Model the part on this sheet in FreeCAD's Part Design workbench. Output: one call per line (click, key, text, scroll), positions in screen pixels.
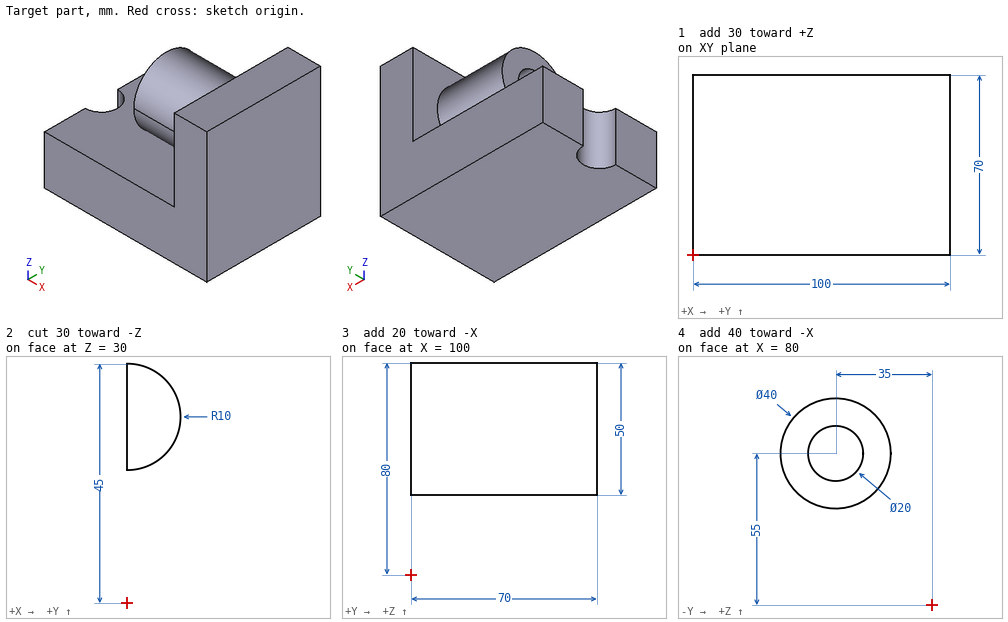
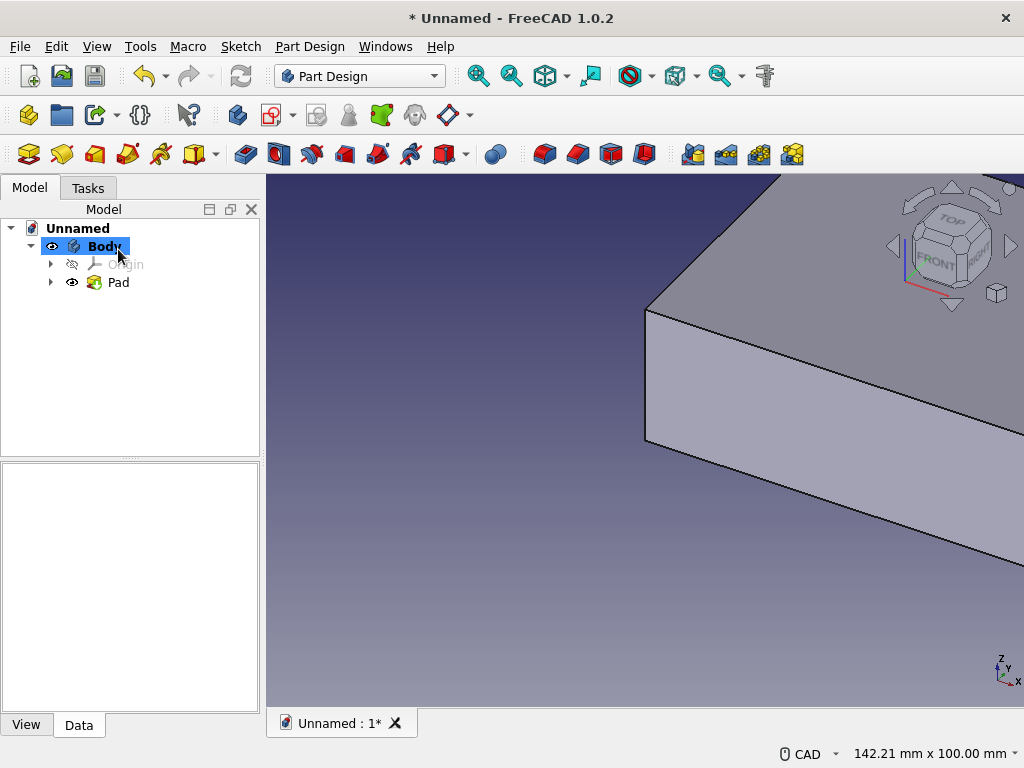
click(479, 76)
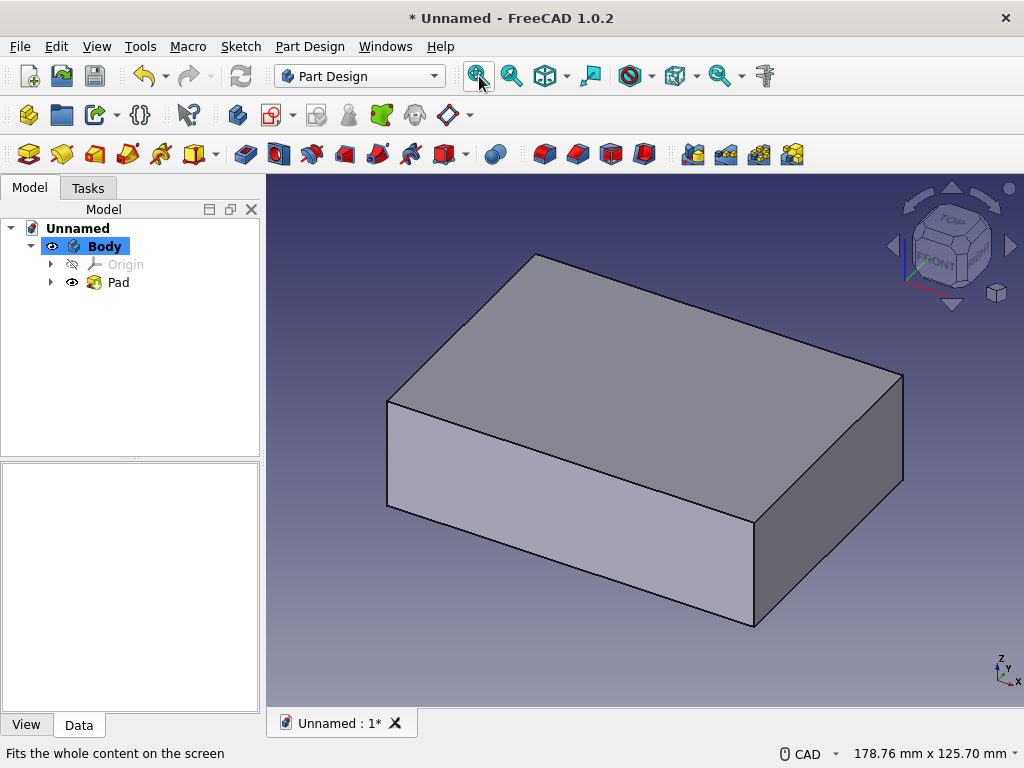
click(697, 405)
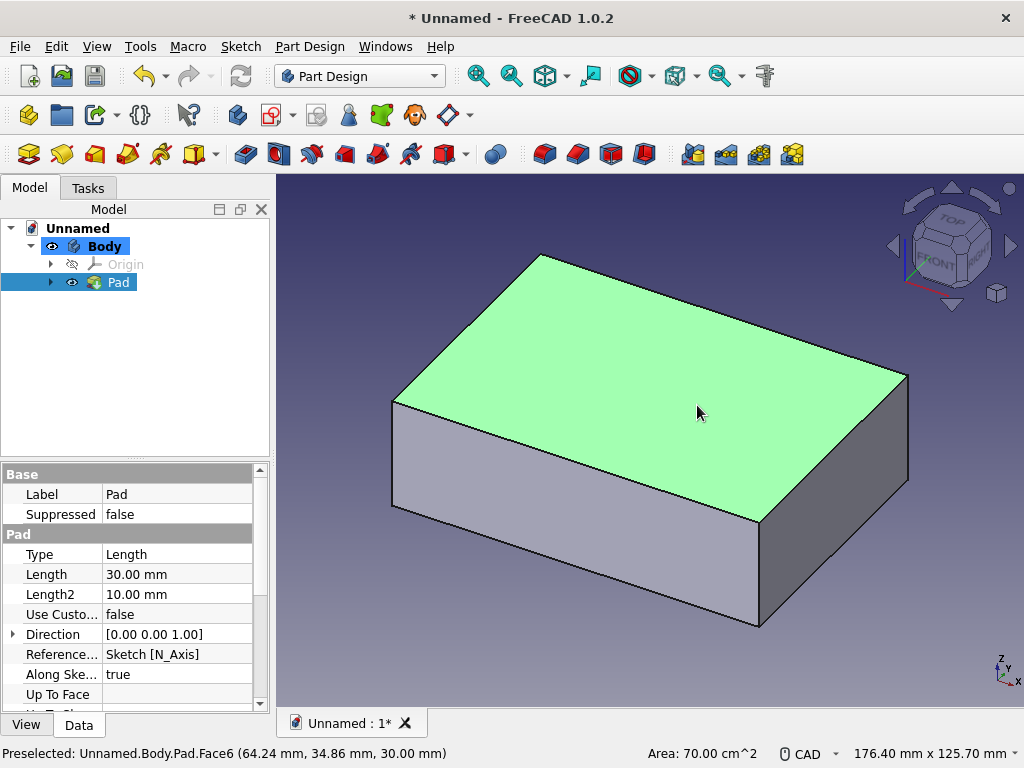
click(270, 116)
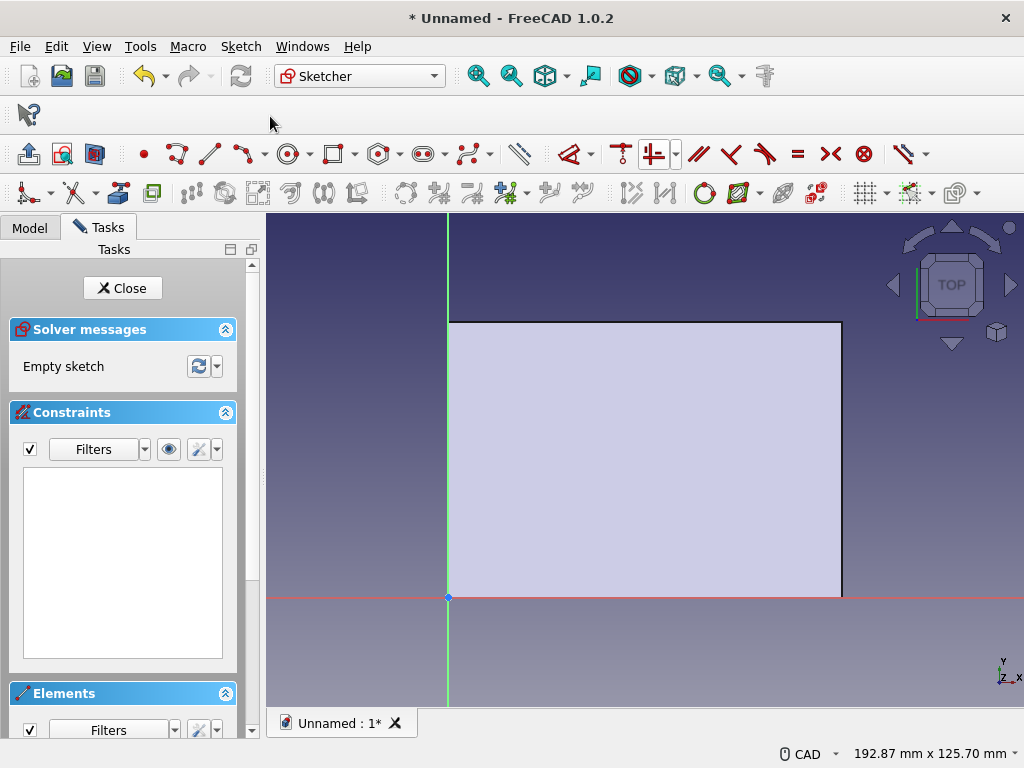
scroll(336, 569, up, 3)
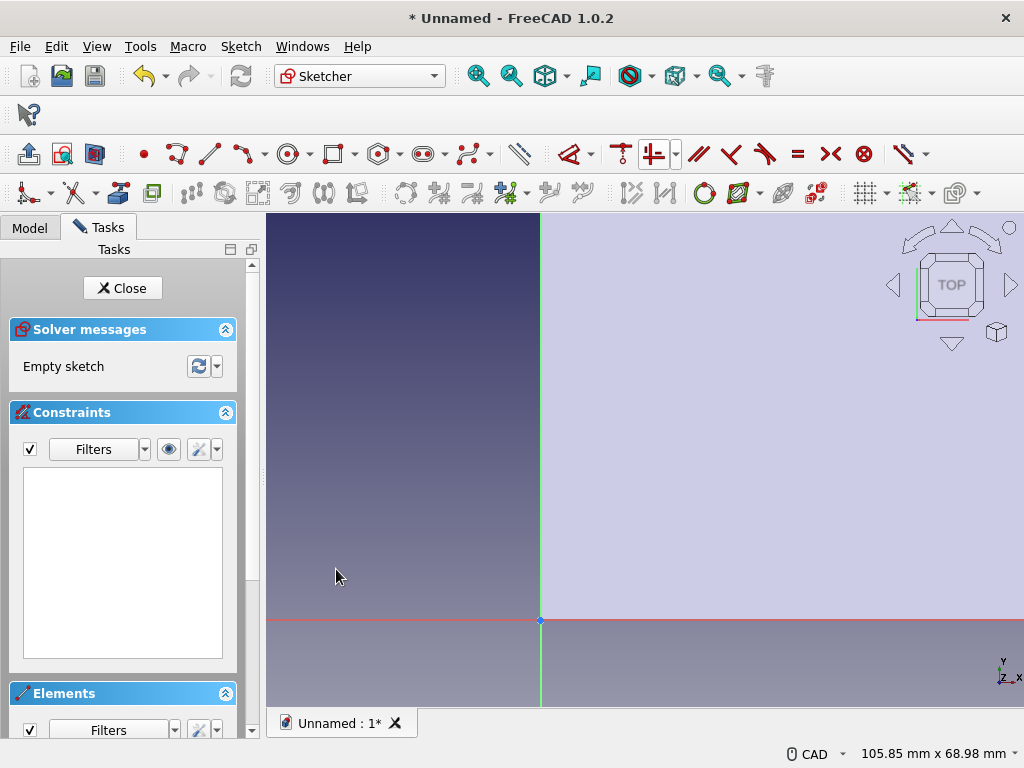
click(210, 154)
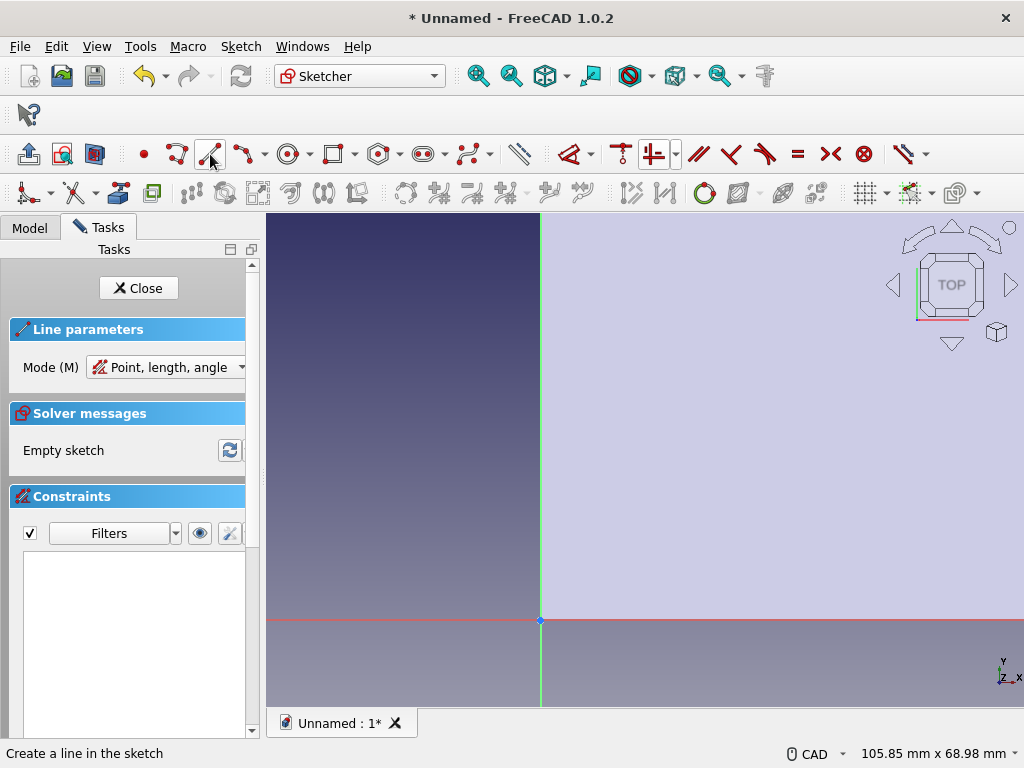
click(541, 298)
click(550, 441)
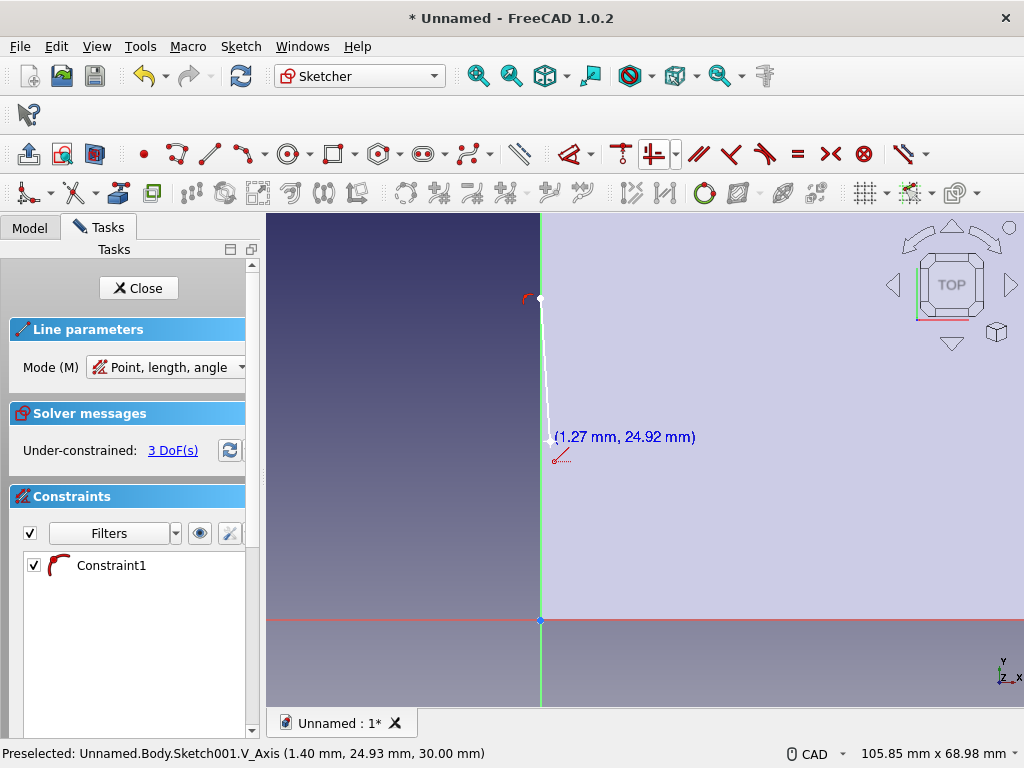
click(242, 154)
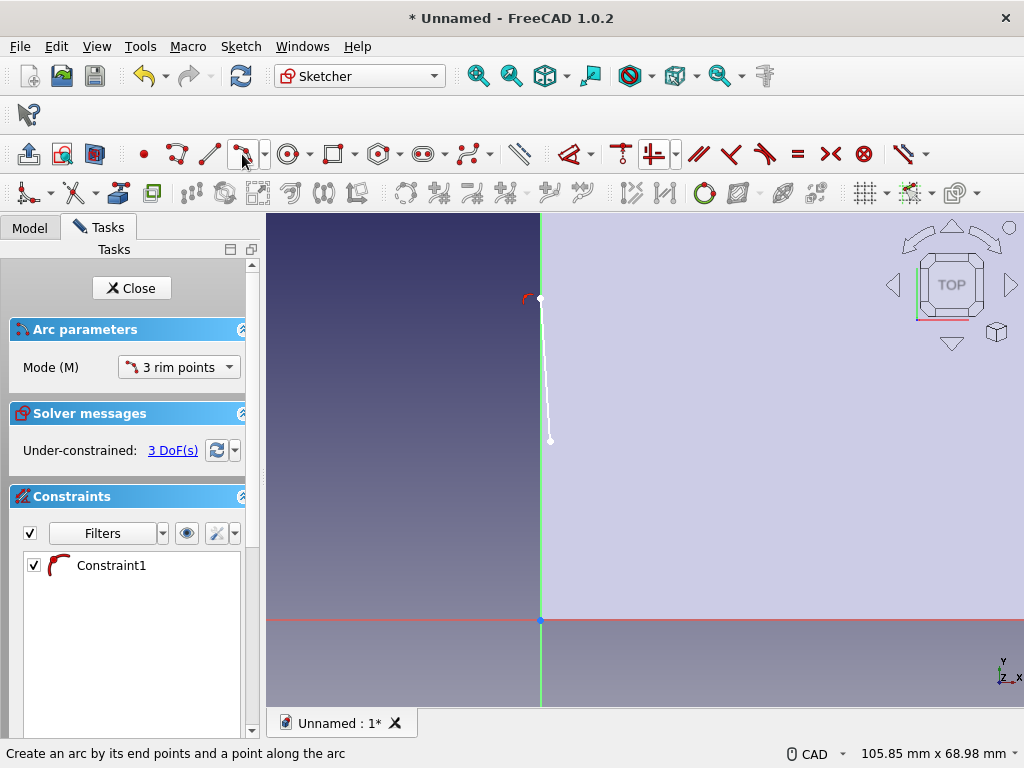
click(550, 442)
click(541, 299)
click(613, 370)
key(Escape)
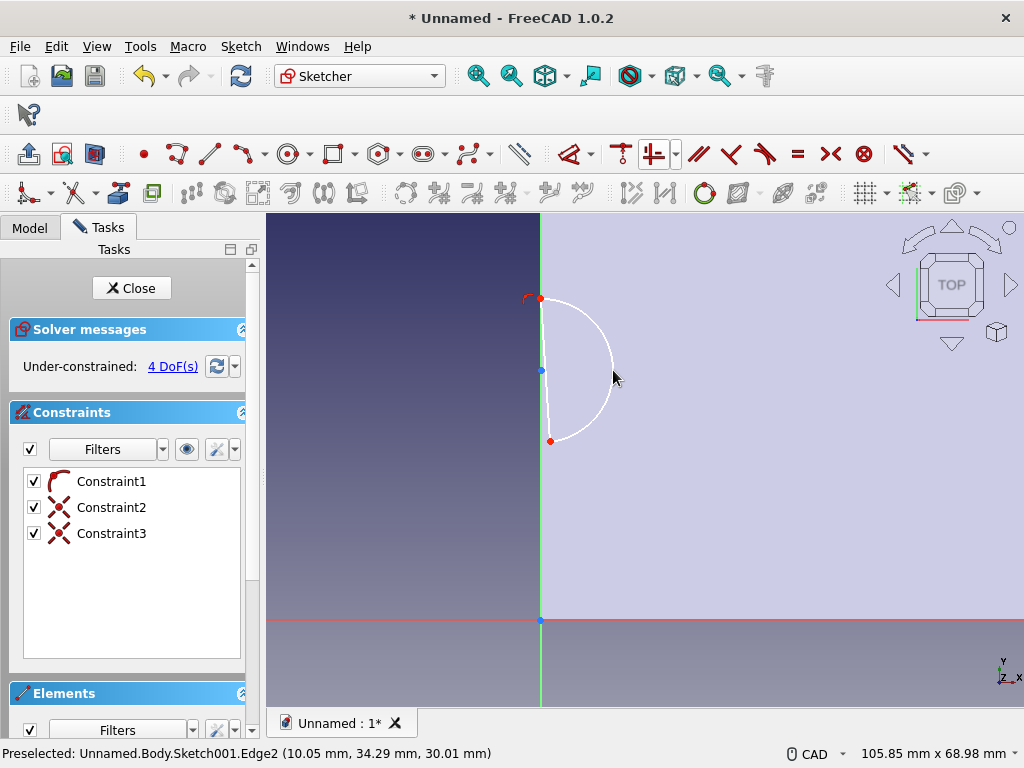
click(544, 342)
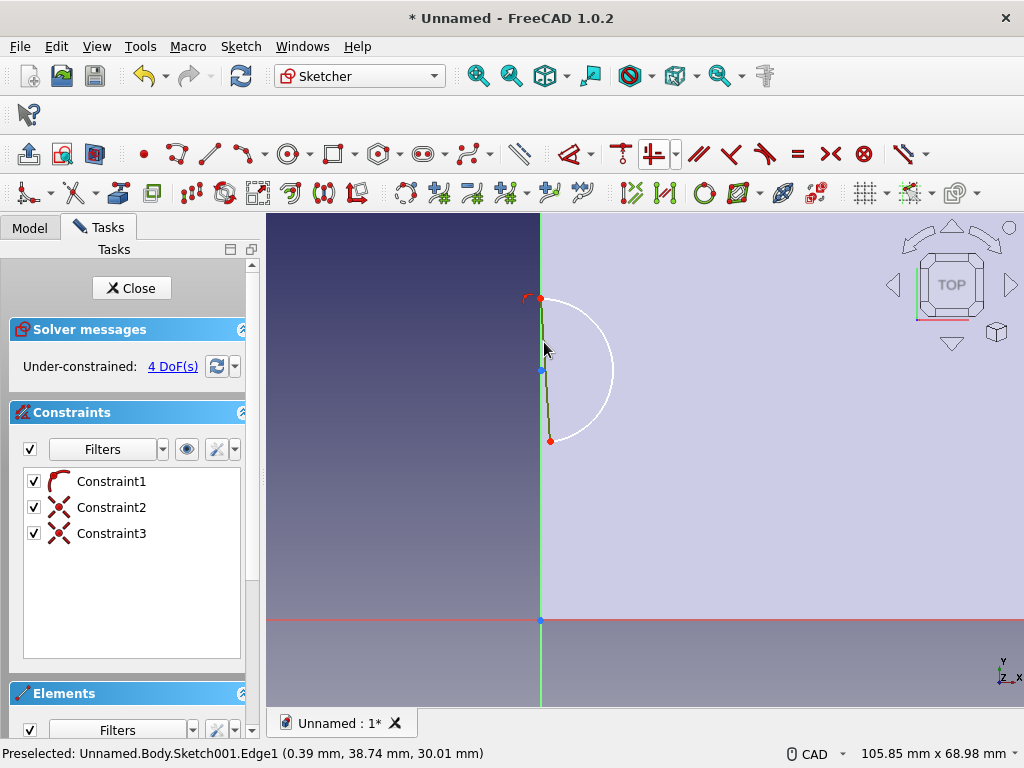
click(676, 154)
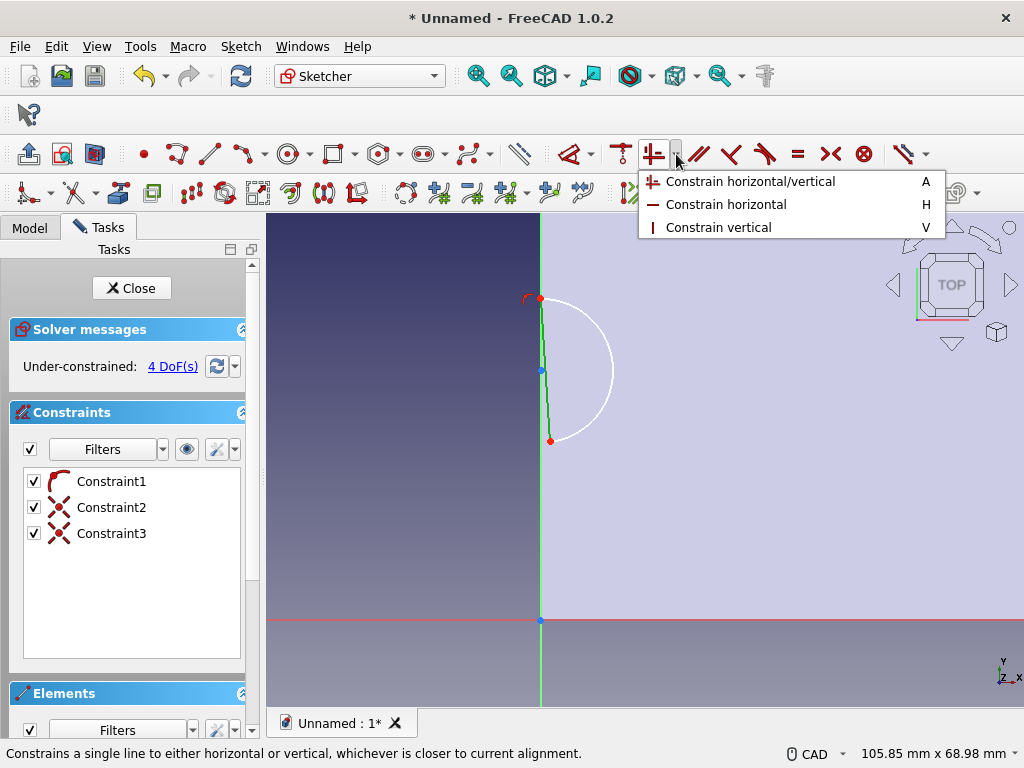
click(792, 228)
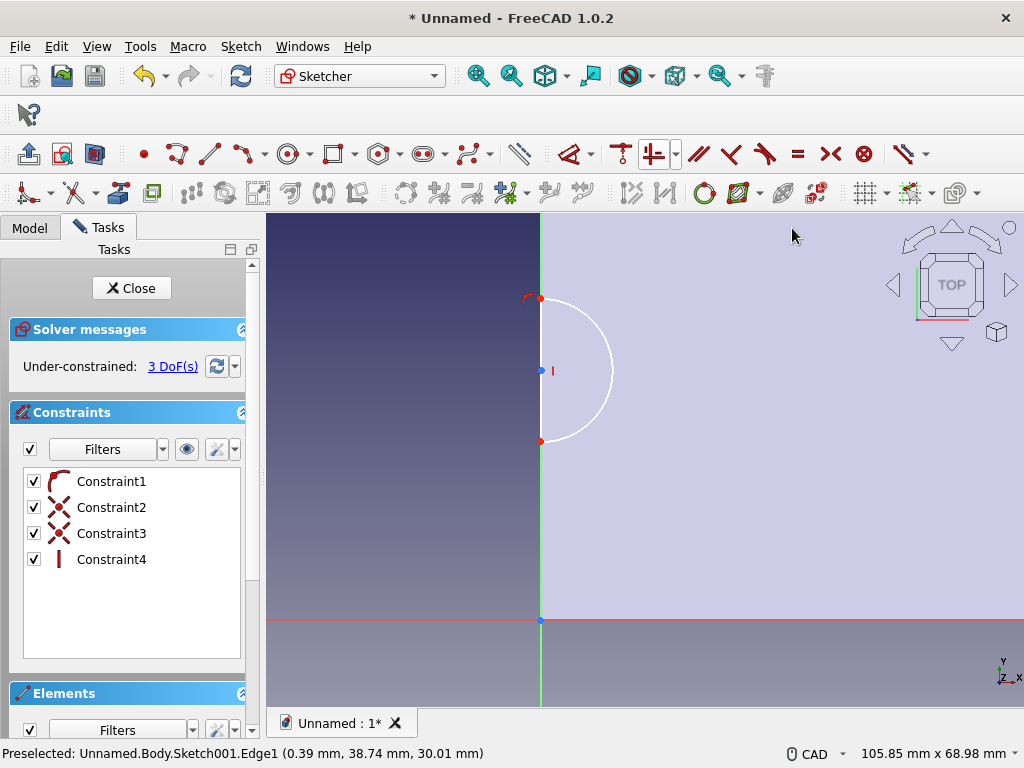
click(541, 370)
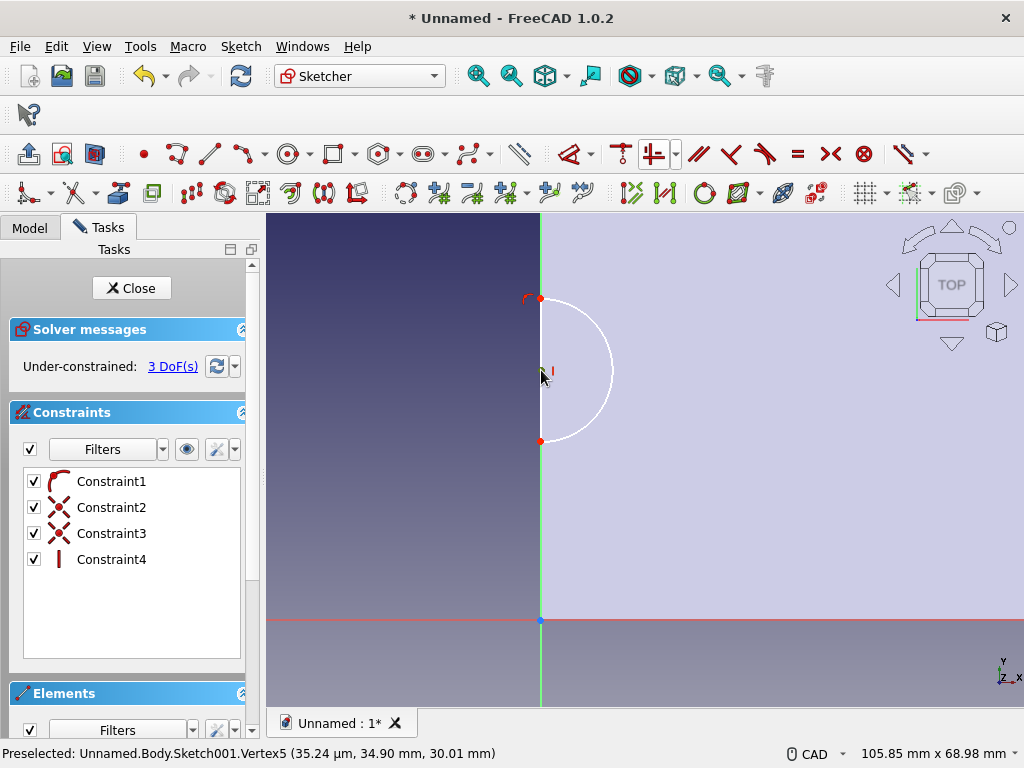
click(541, 585)